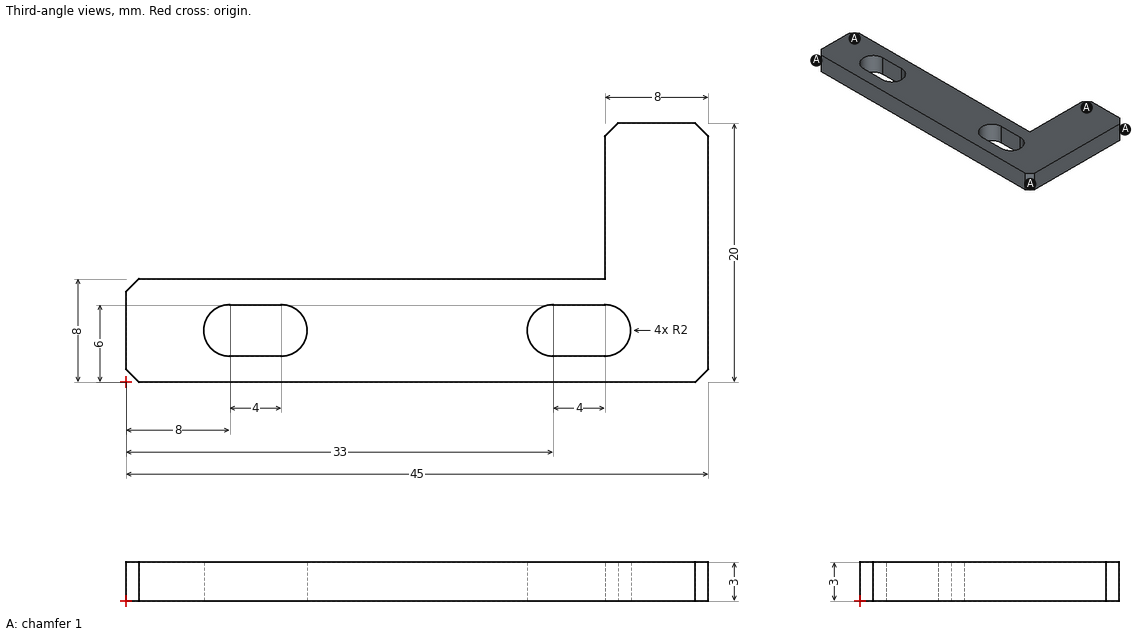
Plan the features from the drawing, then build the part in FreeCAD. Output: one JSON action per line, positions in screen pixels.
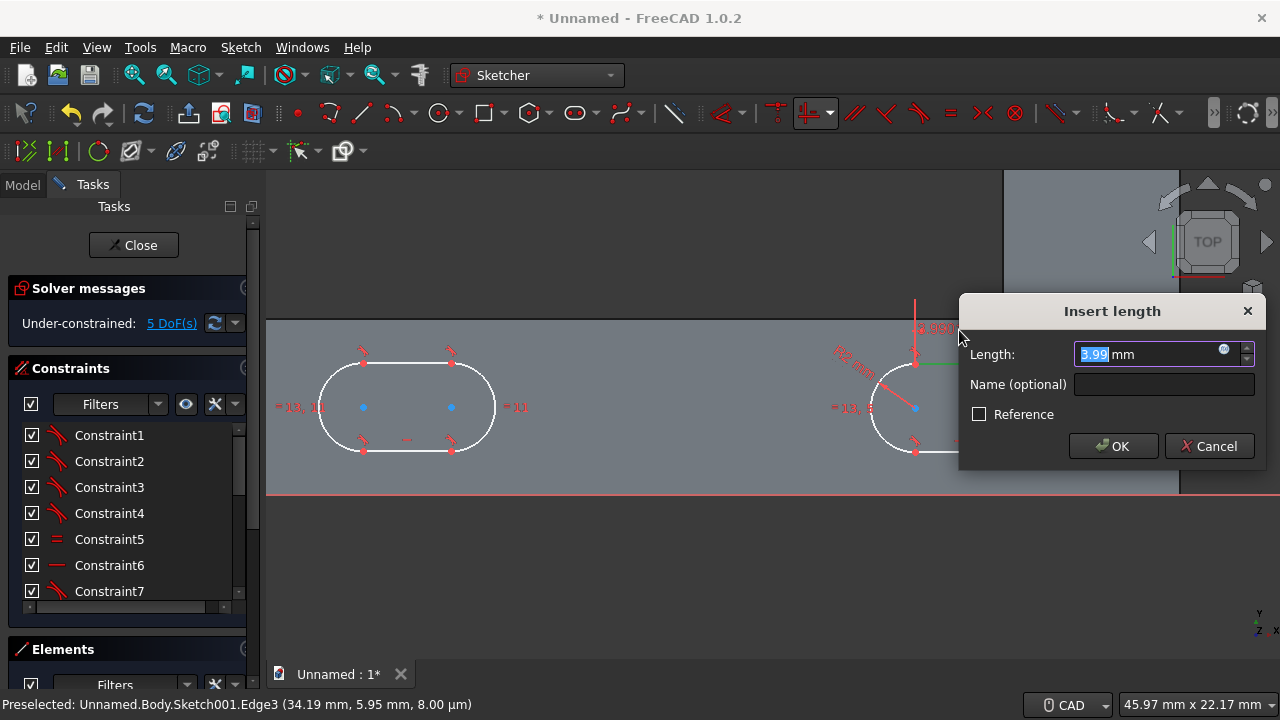
{"action": "type", "text": "4"}
{"action": "key", "text": "Return"}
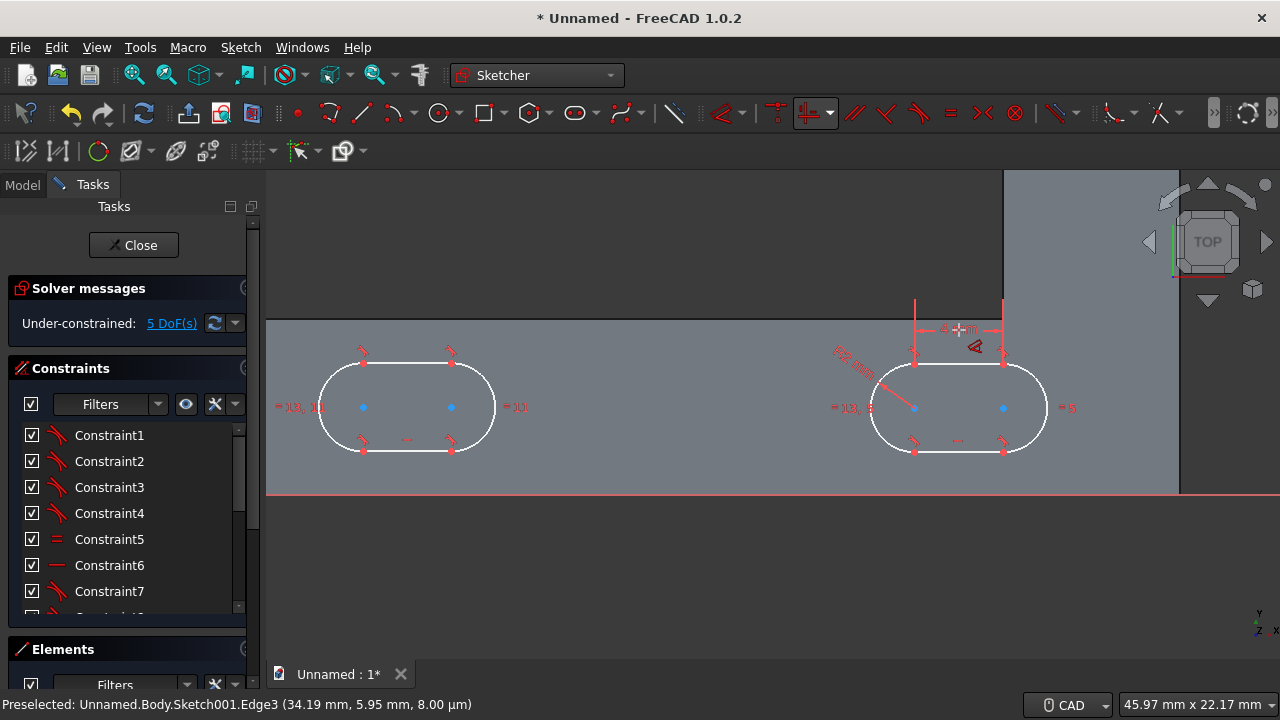
{"action": "left_click", "coordinate": [389, 363]}
{"action": "left_click", "coordinate": [407, 329]}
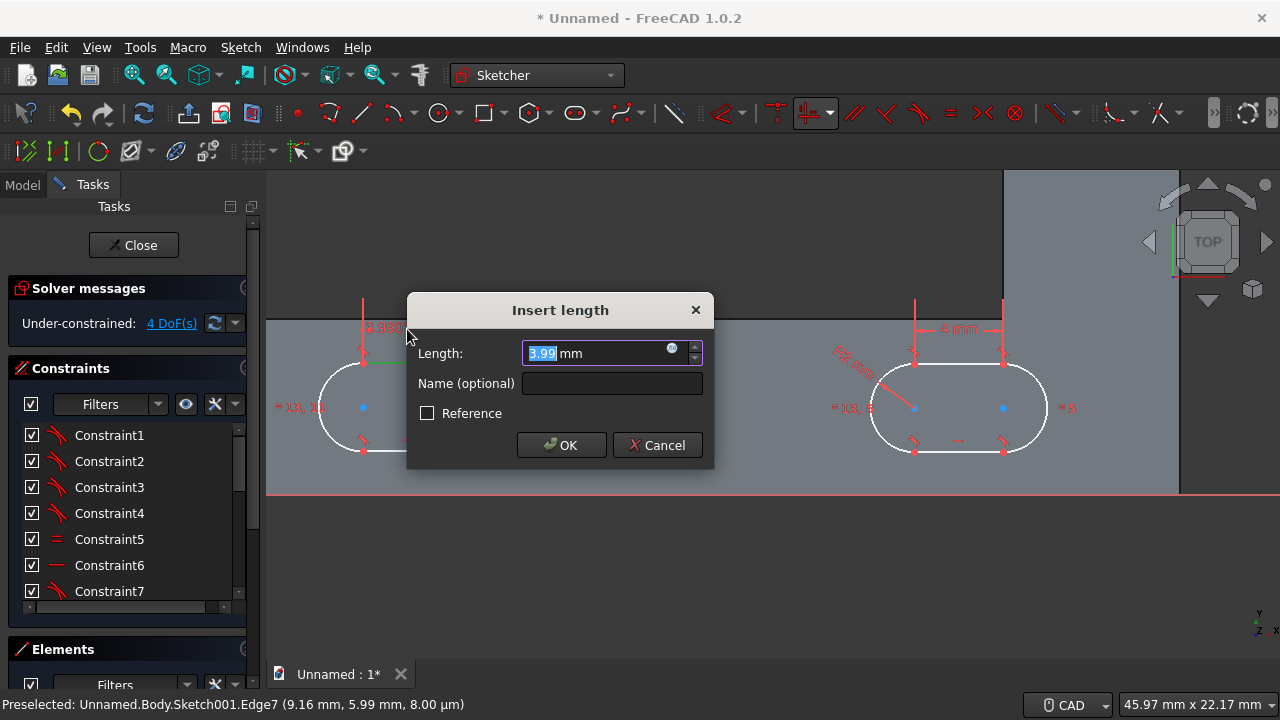
{"action": "type", "text": "4"}
{"action": "key", "text": "Return"}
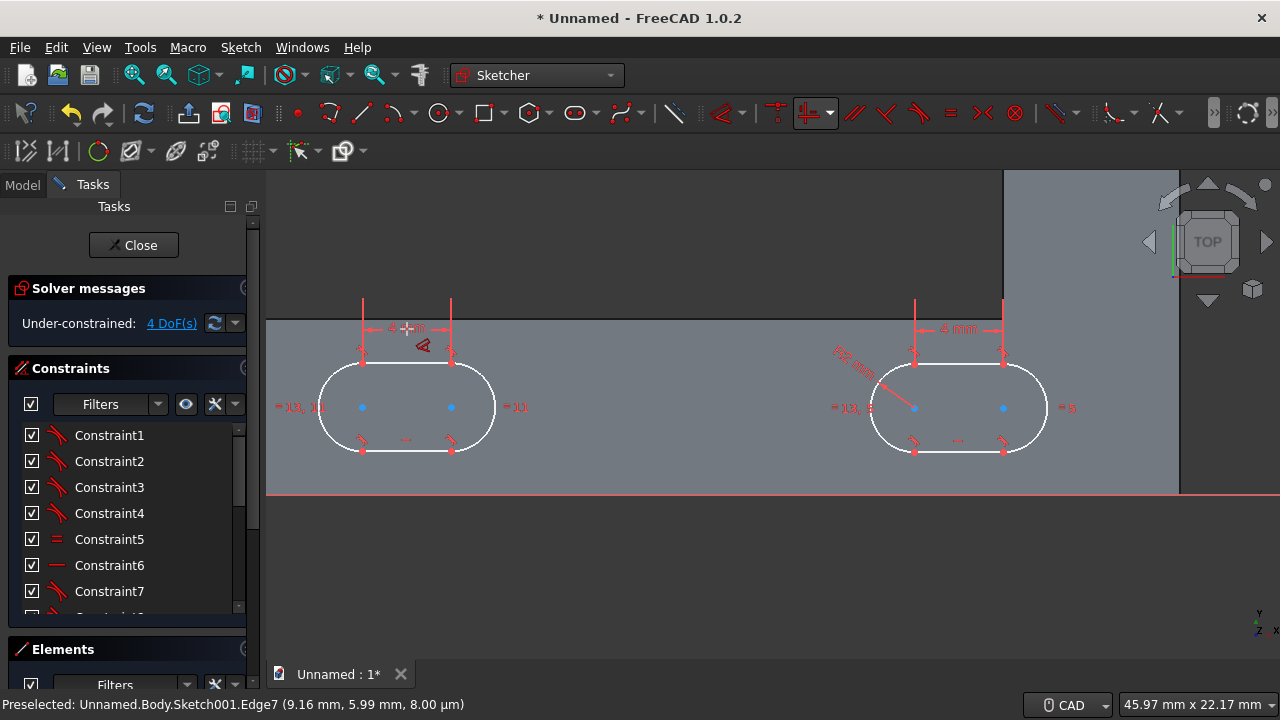
{"action": "left_click", "coordinate": [915, 364]}
{"action": "left_click", "coordinate": [949, 430]}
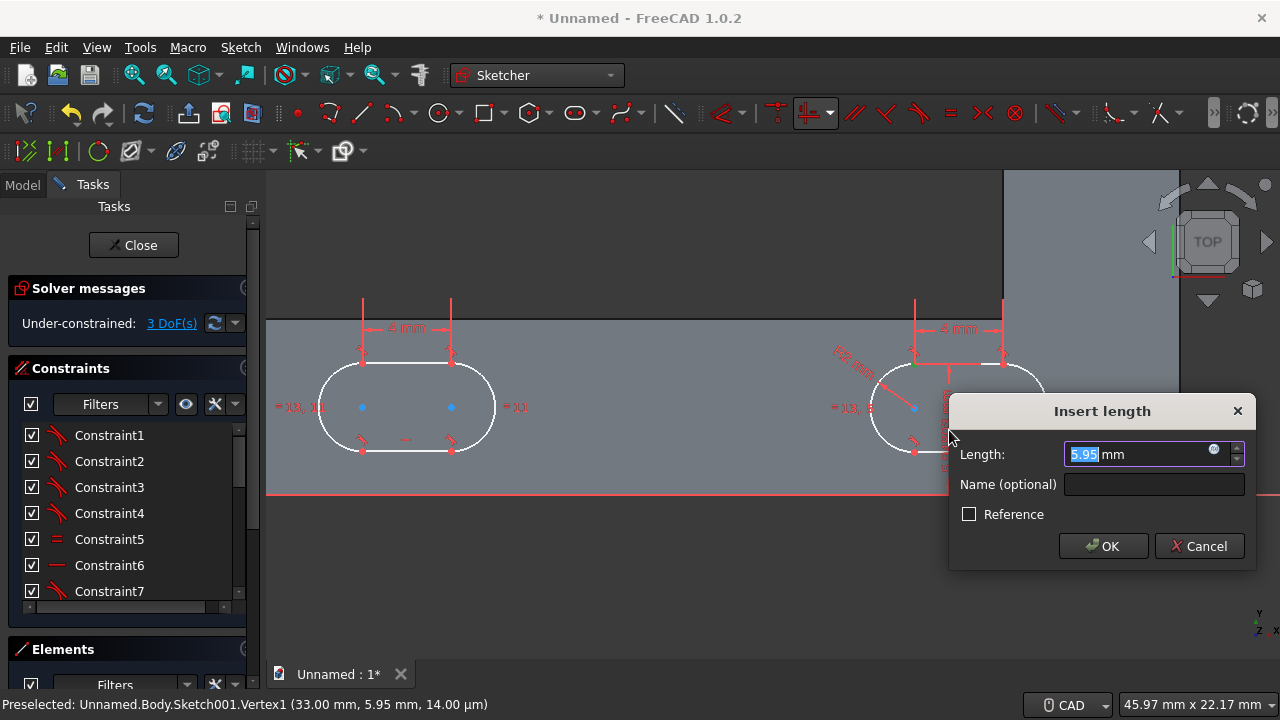
{"action": "type", "text": "6"}
{"action": "key", "text": "Return"}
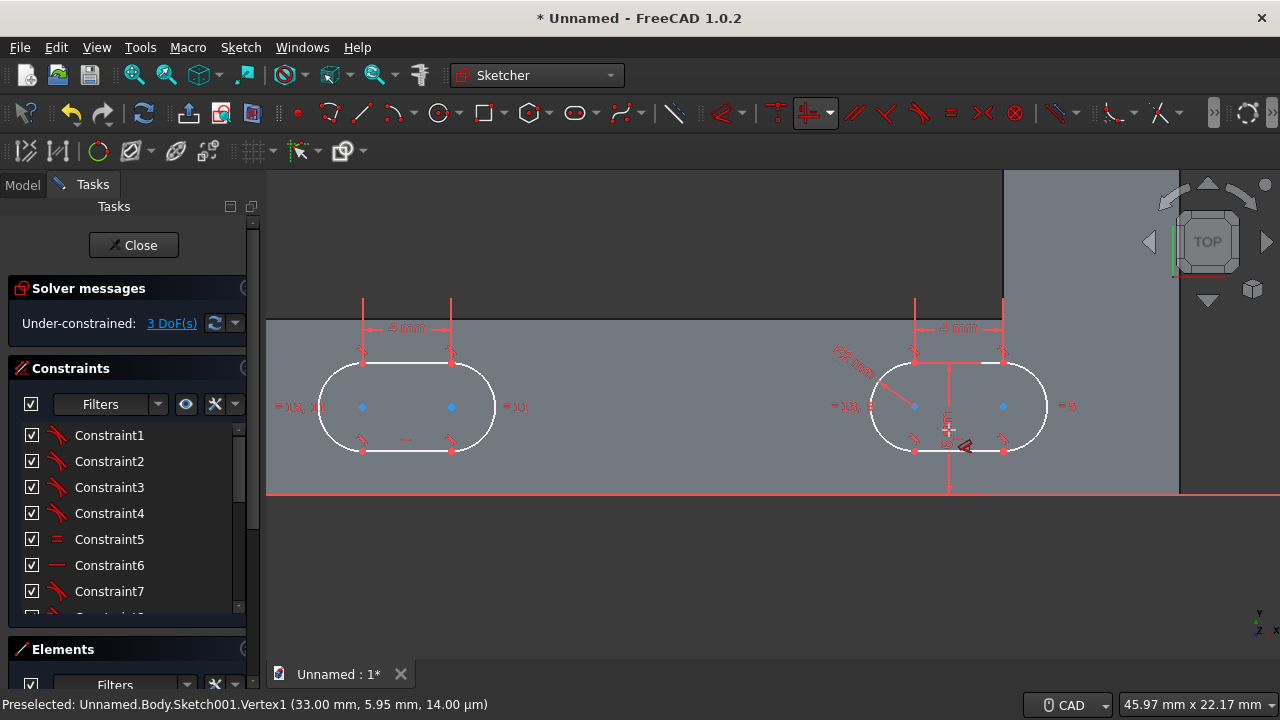
{"action": "left_click", "coordinate": [363, 363]}
{"action": "left_click", "coordinate": [328, 529]}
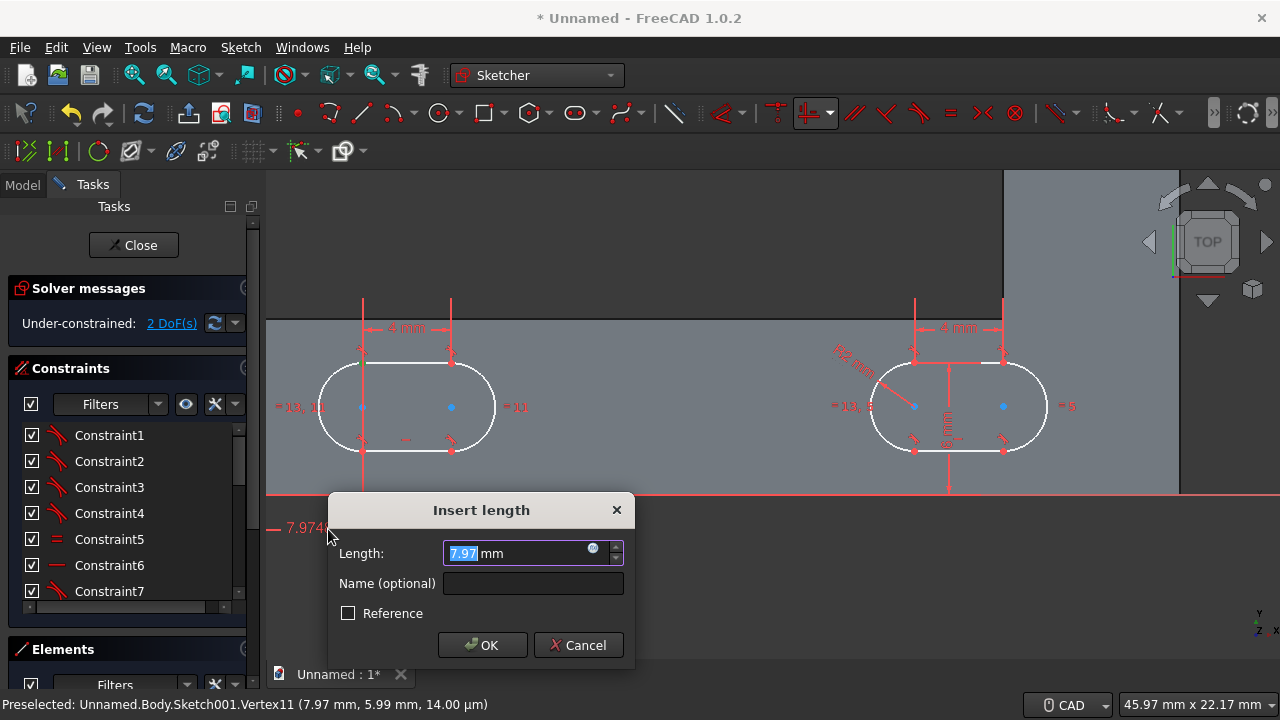
{"action": "type", "text": "8"}
{"action": "key", "text": "Return"}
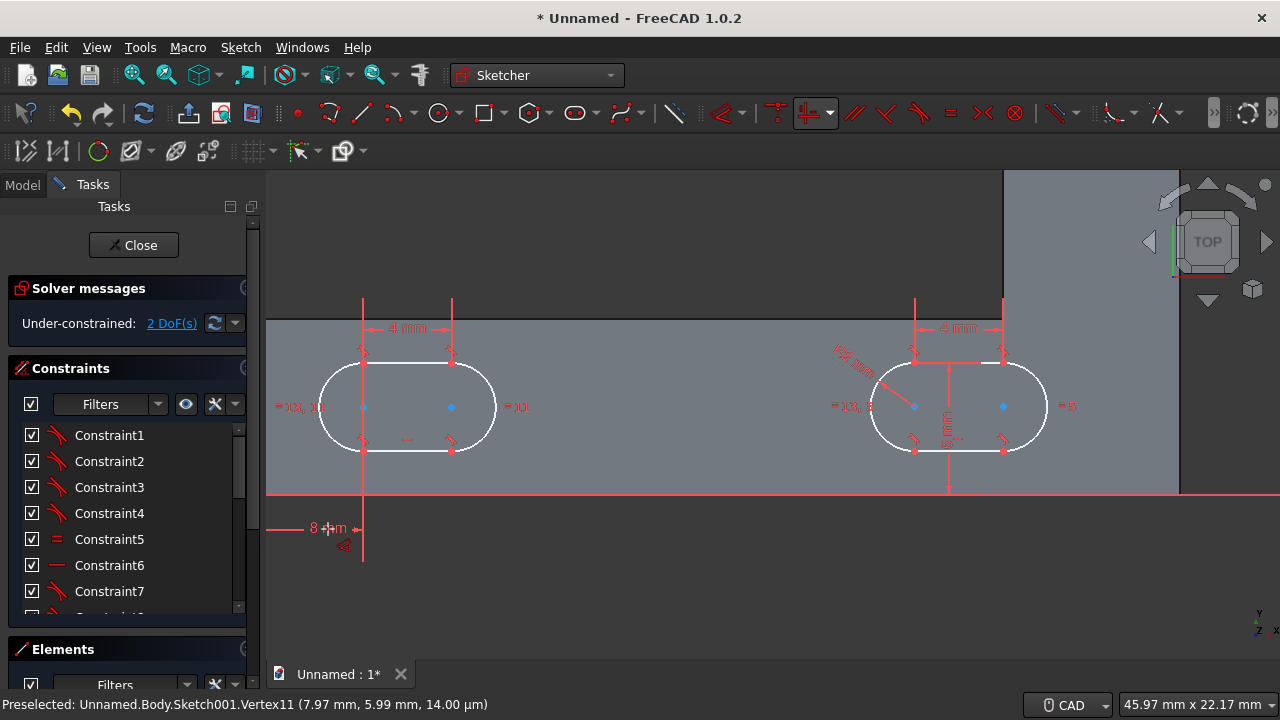
{"action": "left_click", "coordinate": [363, 363]}
{"action": "left_click", "coordinate": [397, 429]}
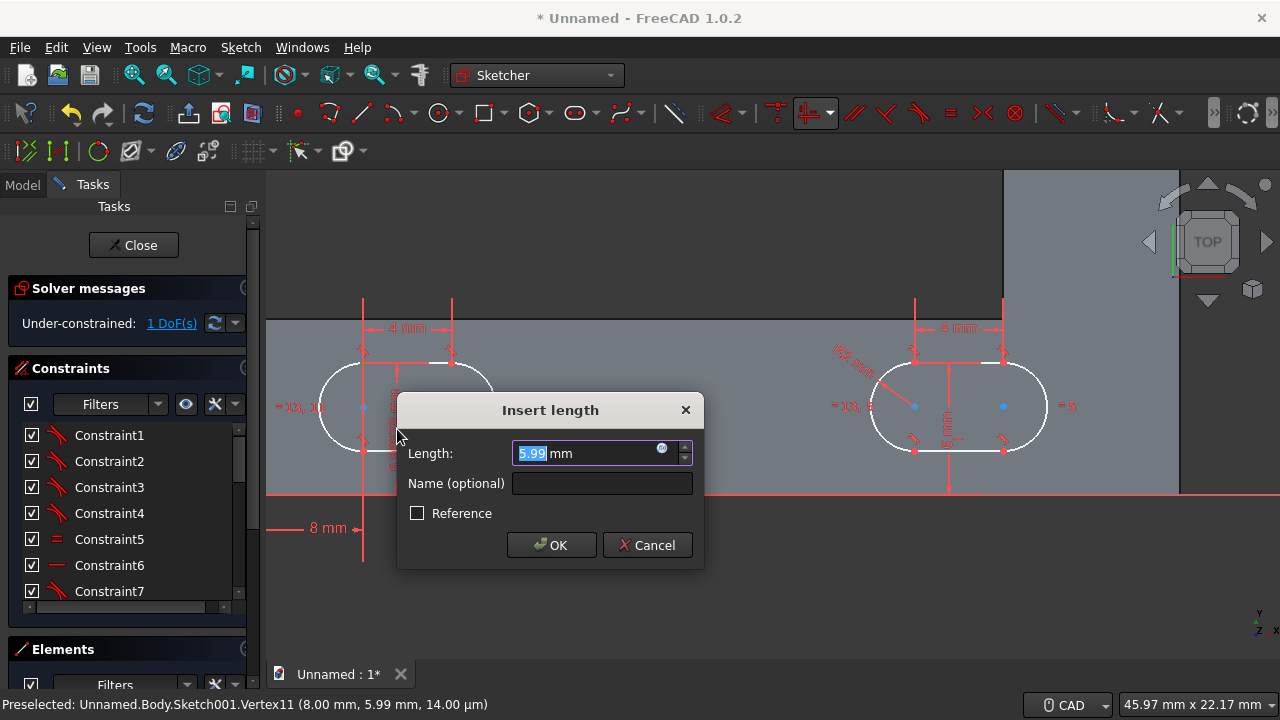
{"action": "type", "text": "6"}
{"action": "key", "text": "Return"}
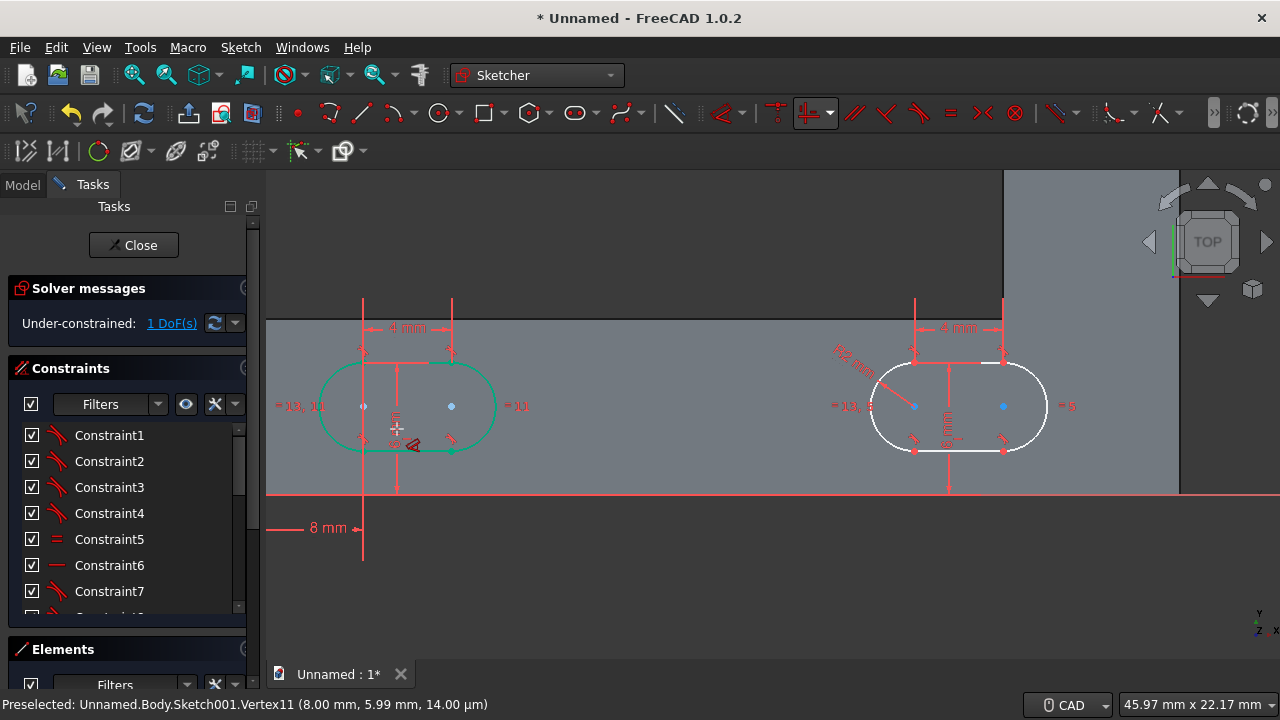
{"action": "left_click", "coordinate": [915, 363]}
{"action": "left_click", "coordinate": [604, 329]}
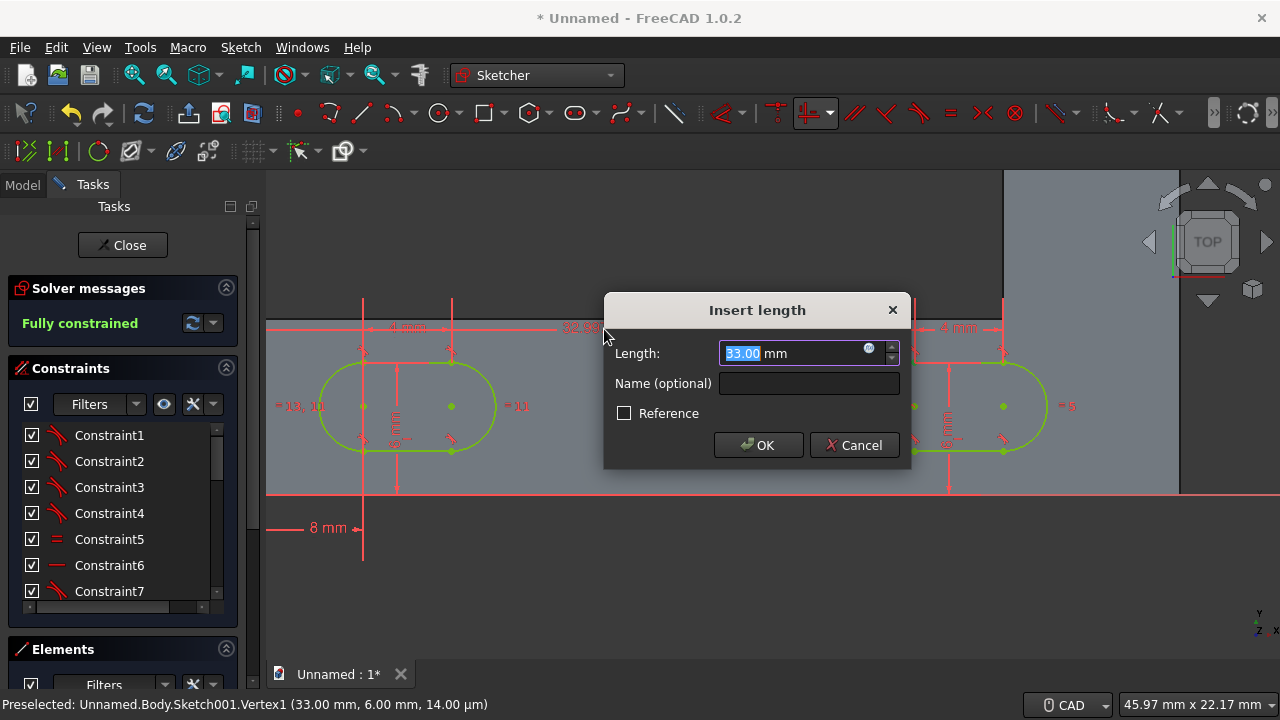
{"action": "type", "text": "33"}
{"action": "key", "text": "Return"}
{"action": "key", "text": "Escape"}